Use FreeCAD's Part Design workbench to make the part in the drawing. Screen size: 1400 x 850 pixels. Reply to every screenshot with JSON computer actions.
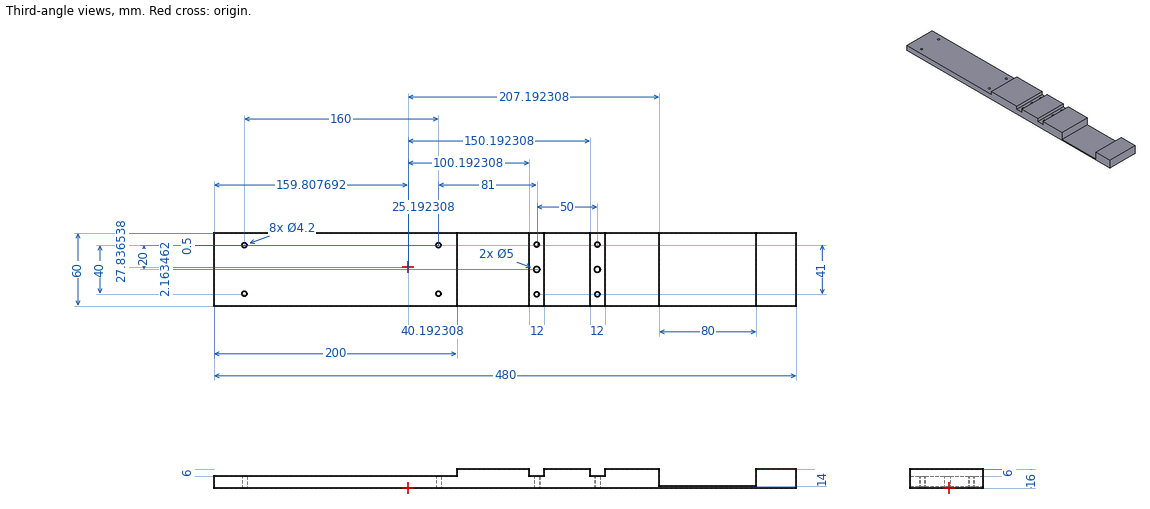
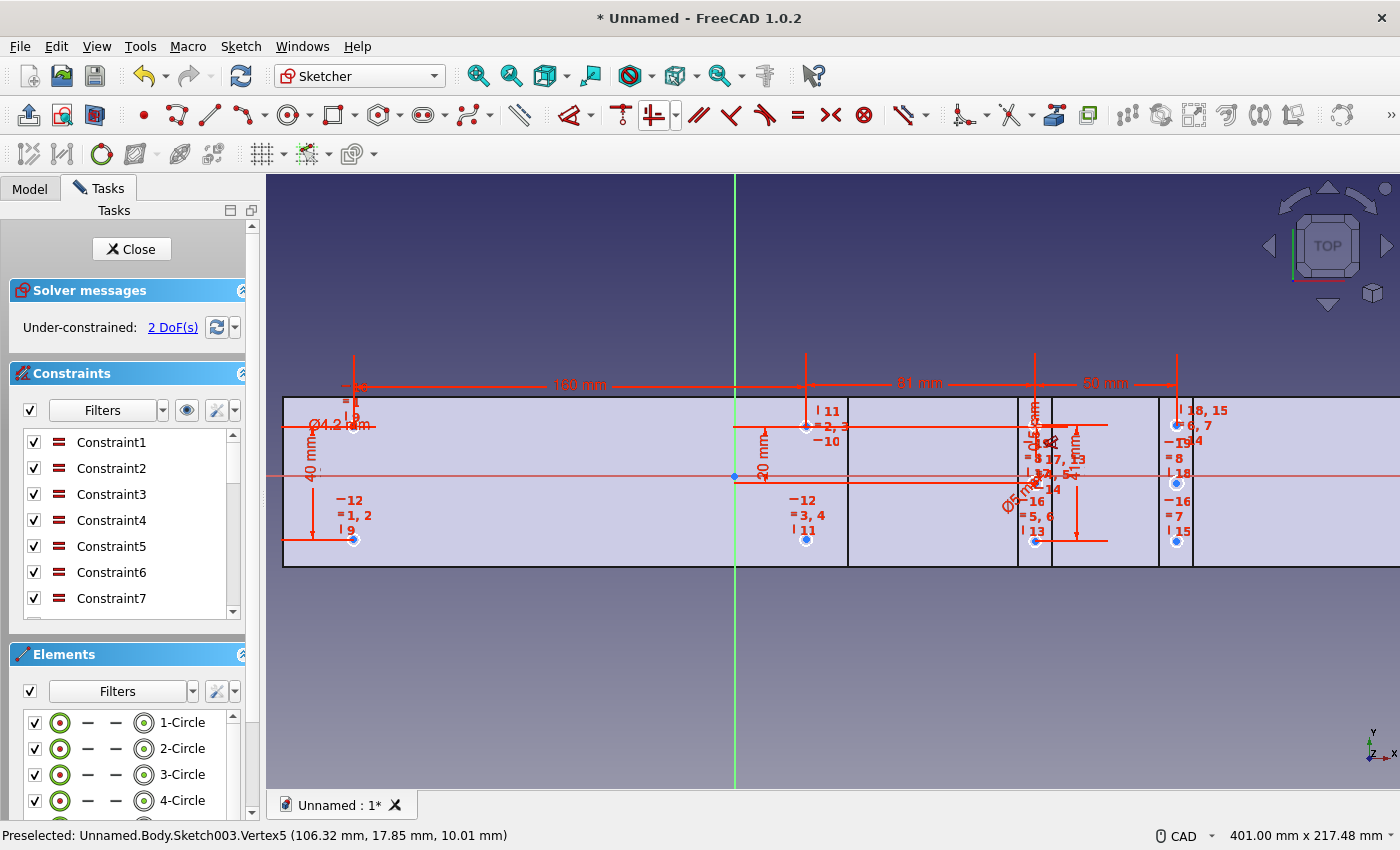
{"action": "scroll", "coordinate": [1035, 483], "scroll_direction": "up", "scroll_amount": 10}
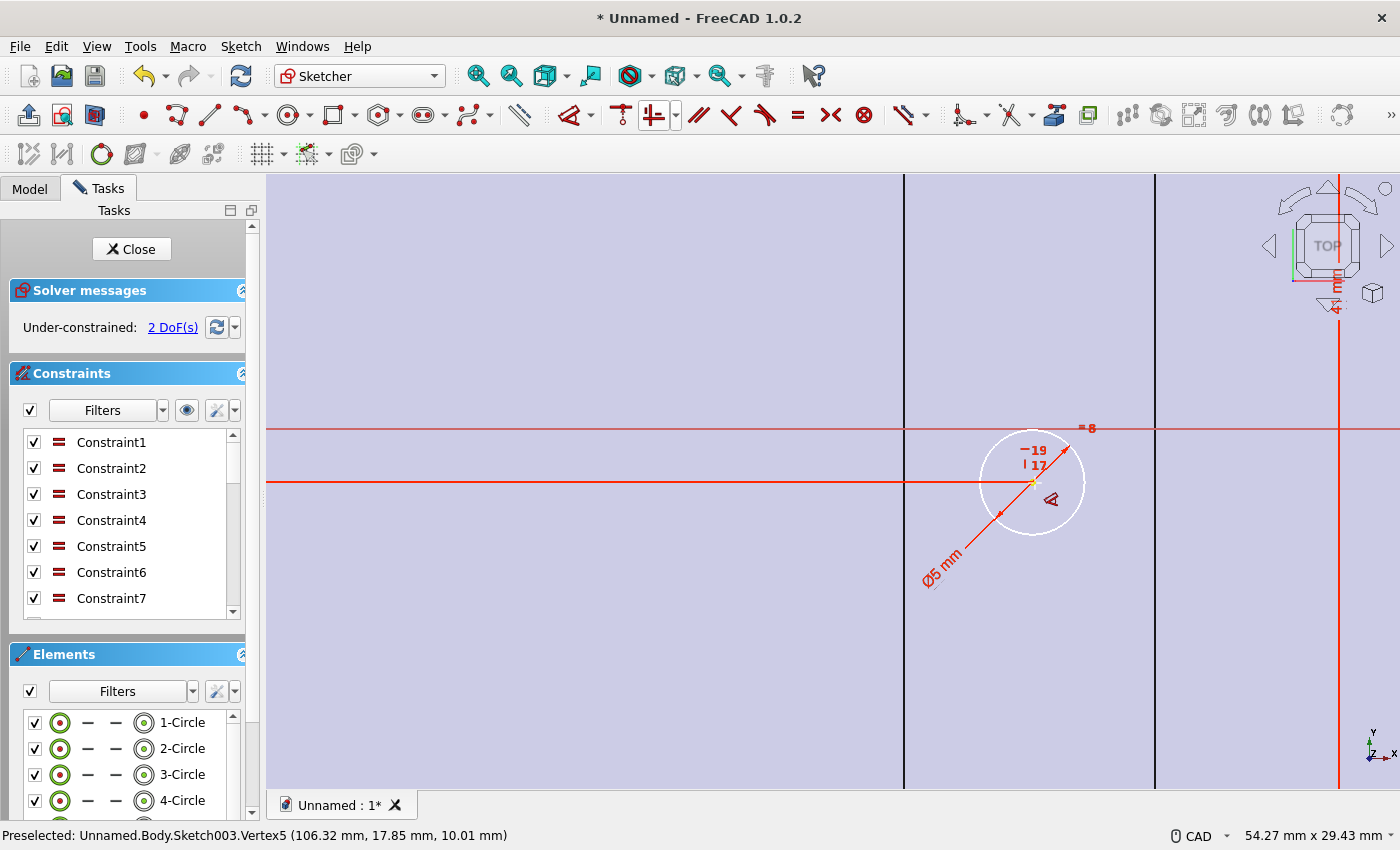
{"action": "left_click", "coordinate": [1032, 482]}
{"action": "left_click", "coordinate": [1066, 468]}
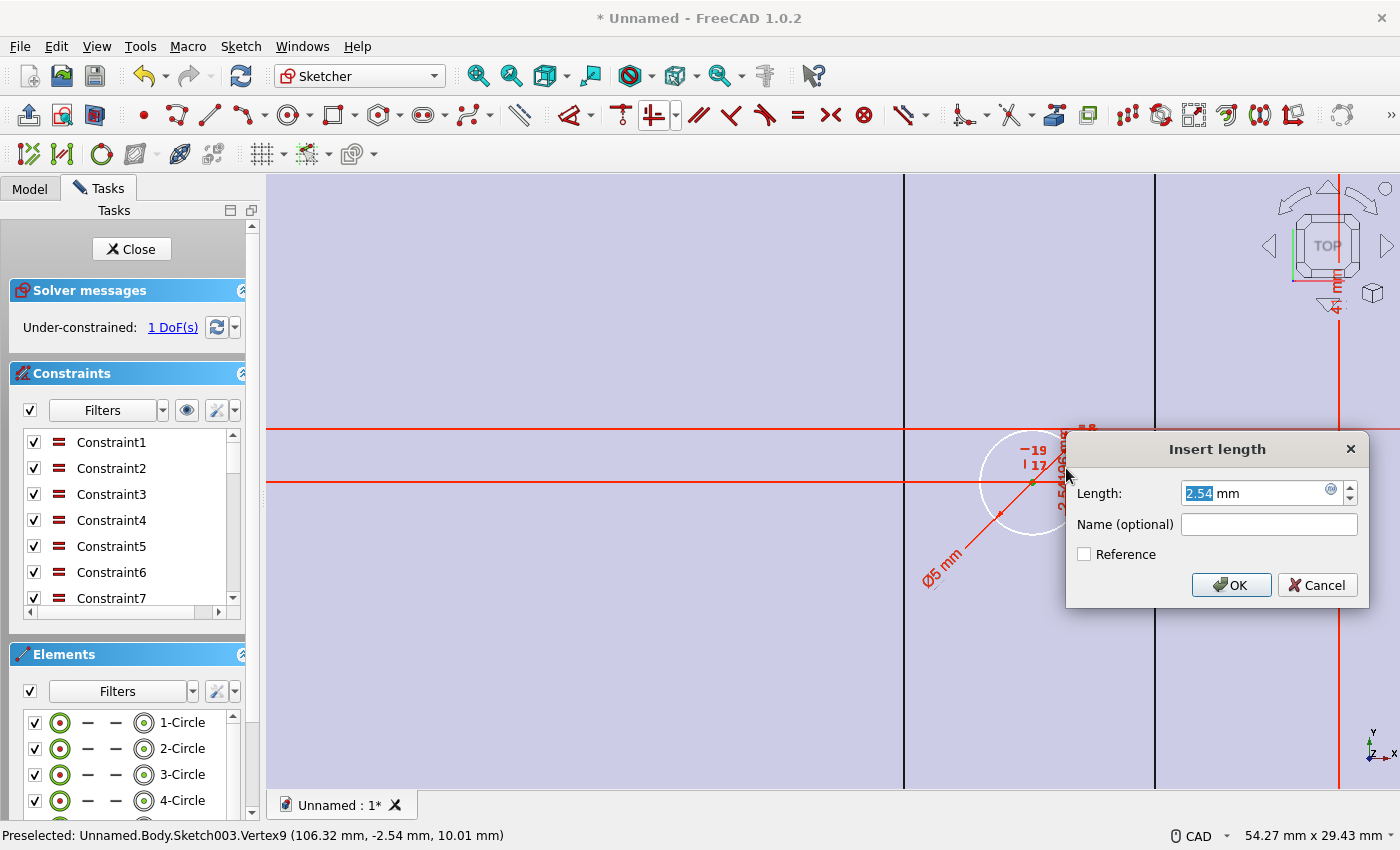
{"action": "type", "text": "2.163462"}
{"action": "key", "text": "Return"}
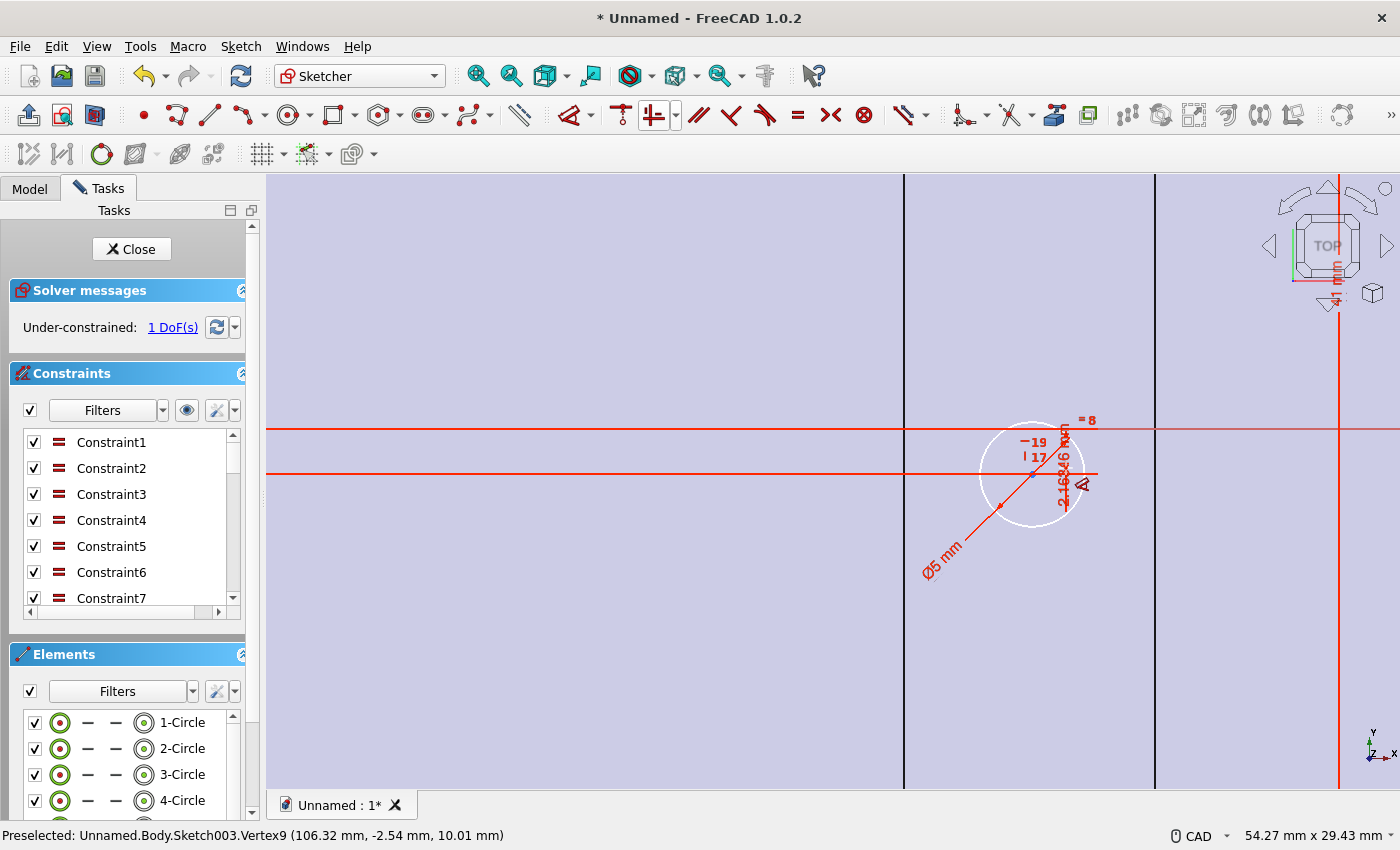
{"action": "scroll", "coordinate": [980, 482], "scroll_direction": "down", "scroll_amount": 11}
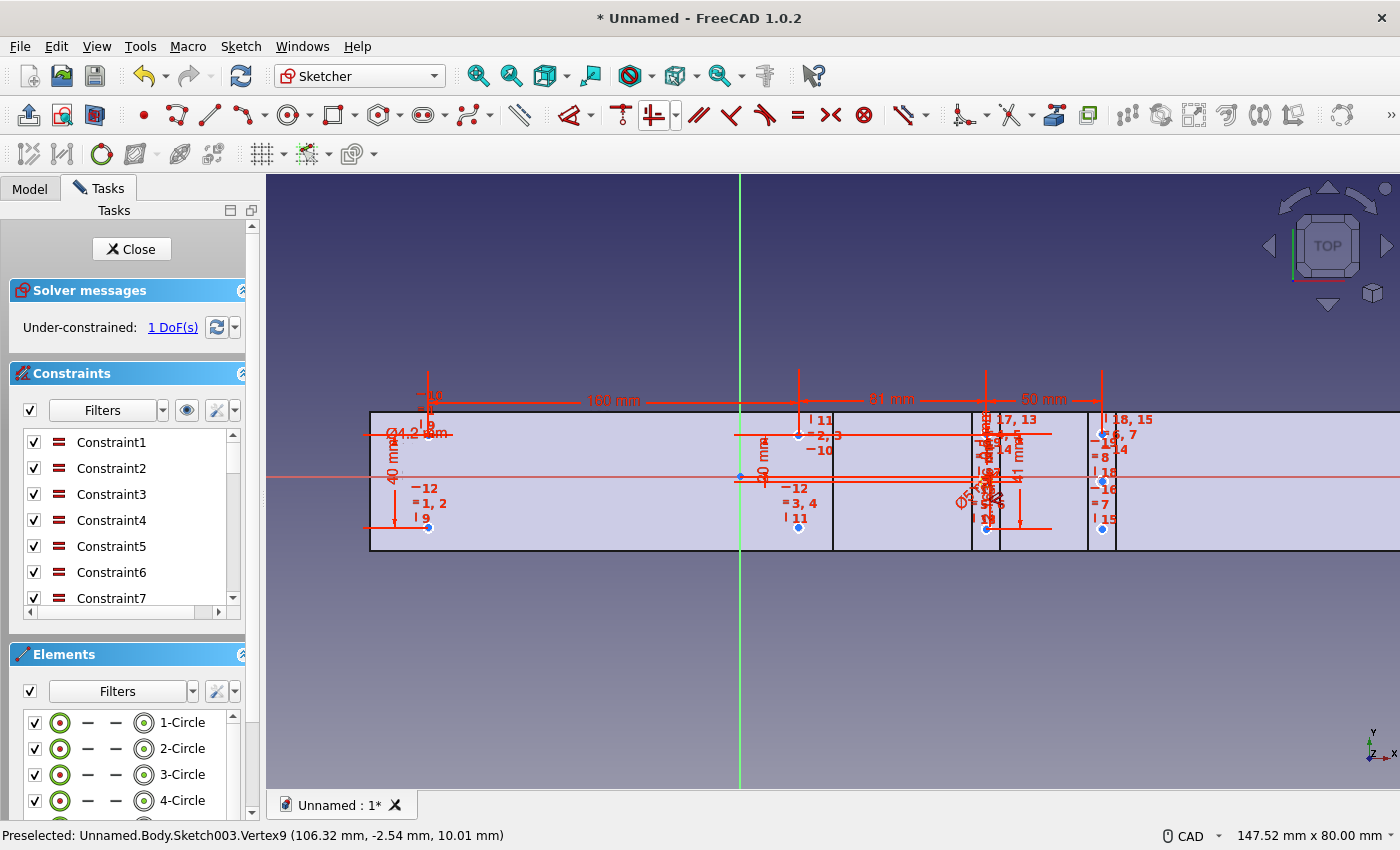
{"action": "left_click", "coordinate": [799, 435]}
{"action": "left_click", "coordinate": [770, 401]}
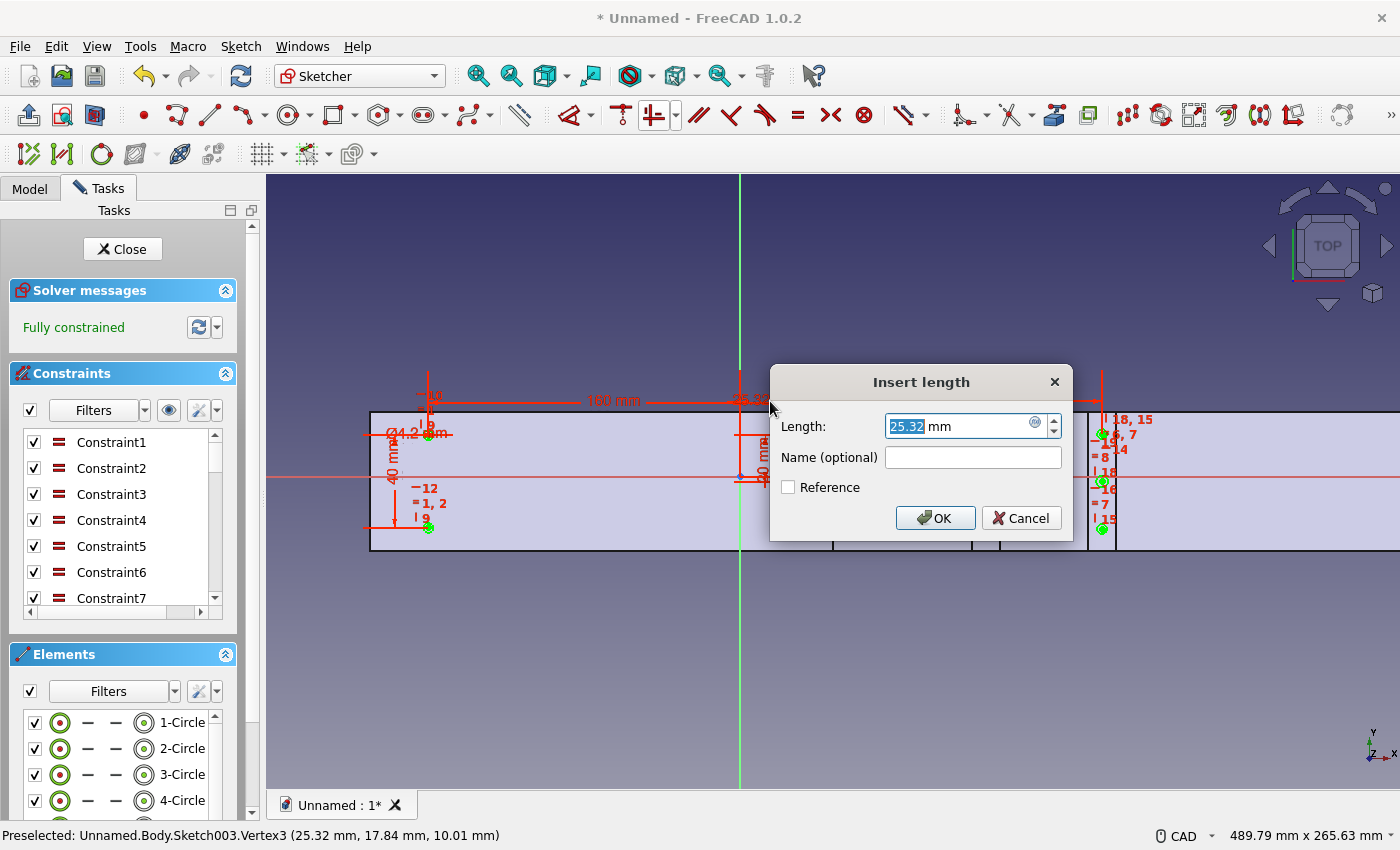
{"action": "type", "text": "25.192308"}
{"action": "key", "text": "Return"}
{"action": "key", "text": "Escape"}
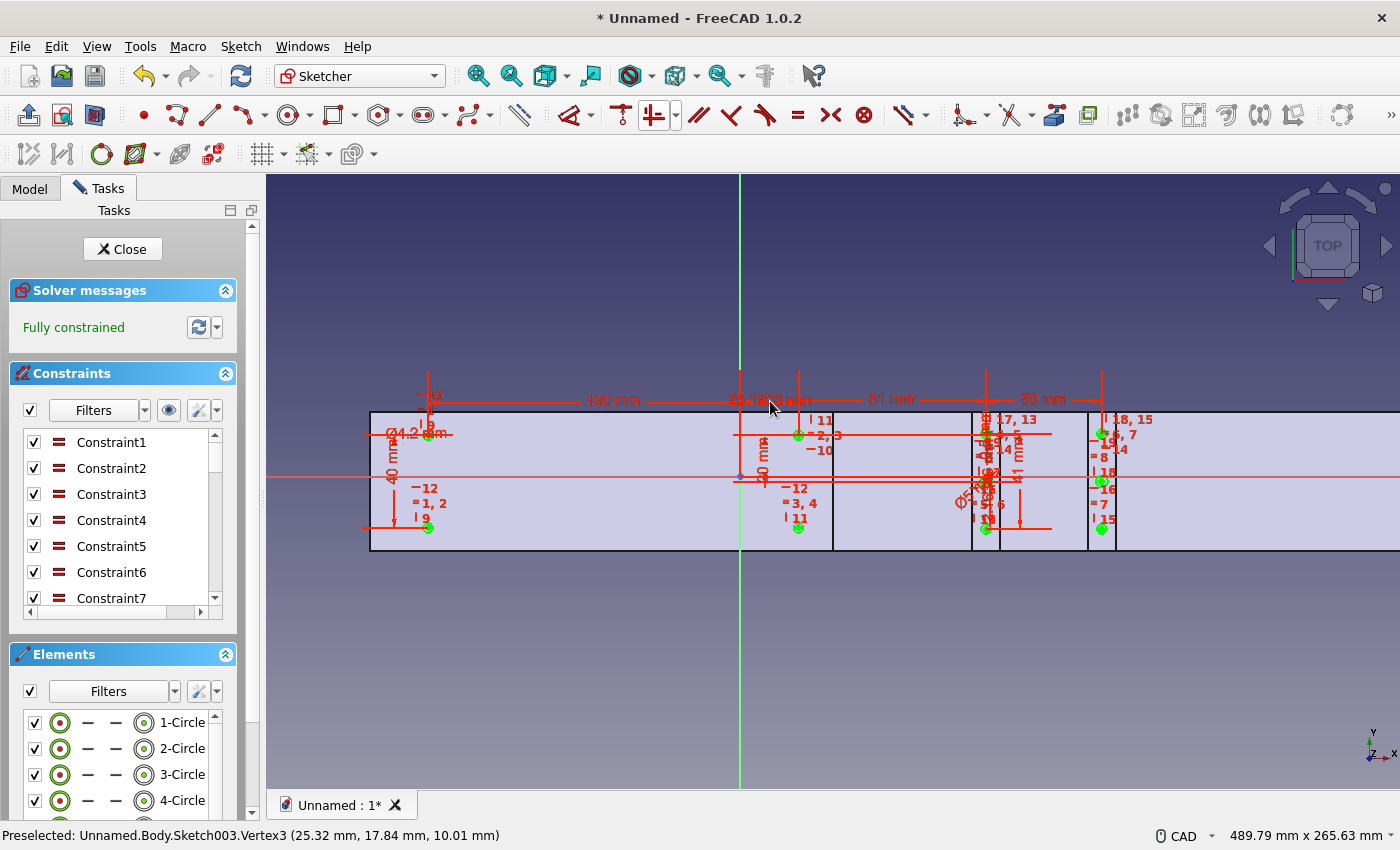
{"action": "left_click", "coordinate": [123, 249]}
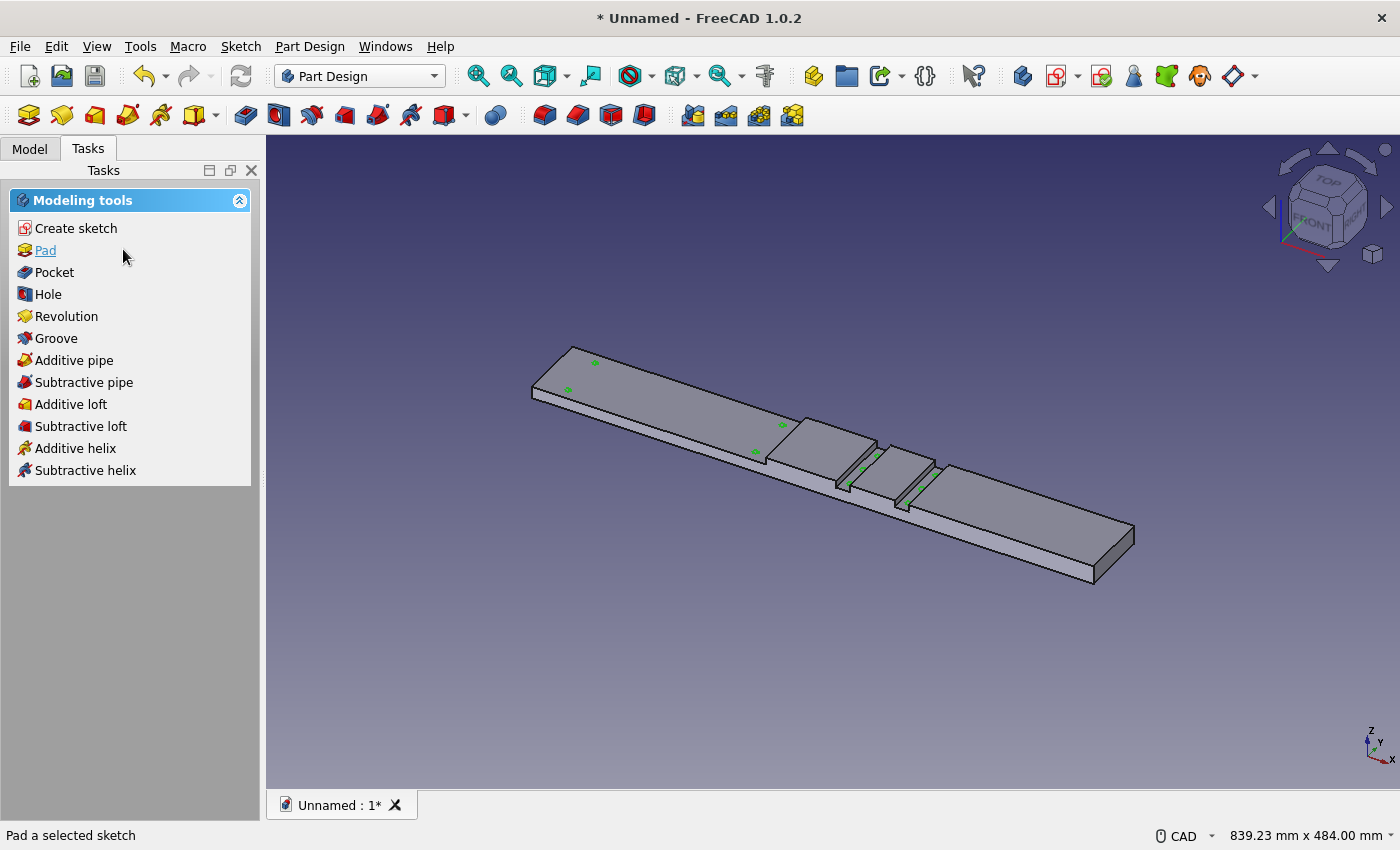
{"action": "left_click", "coordinate": [246, 116]}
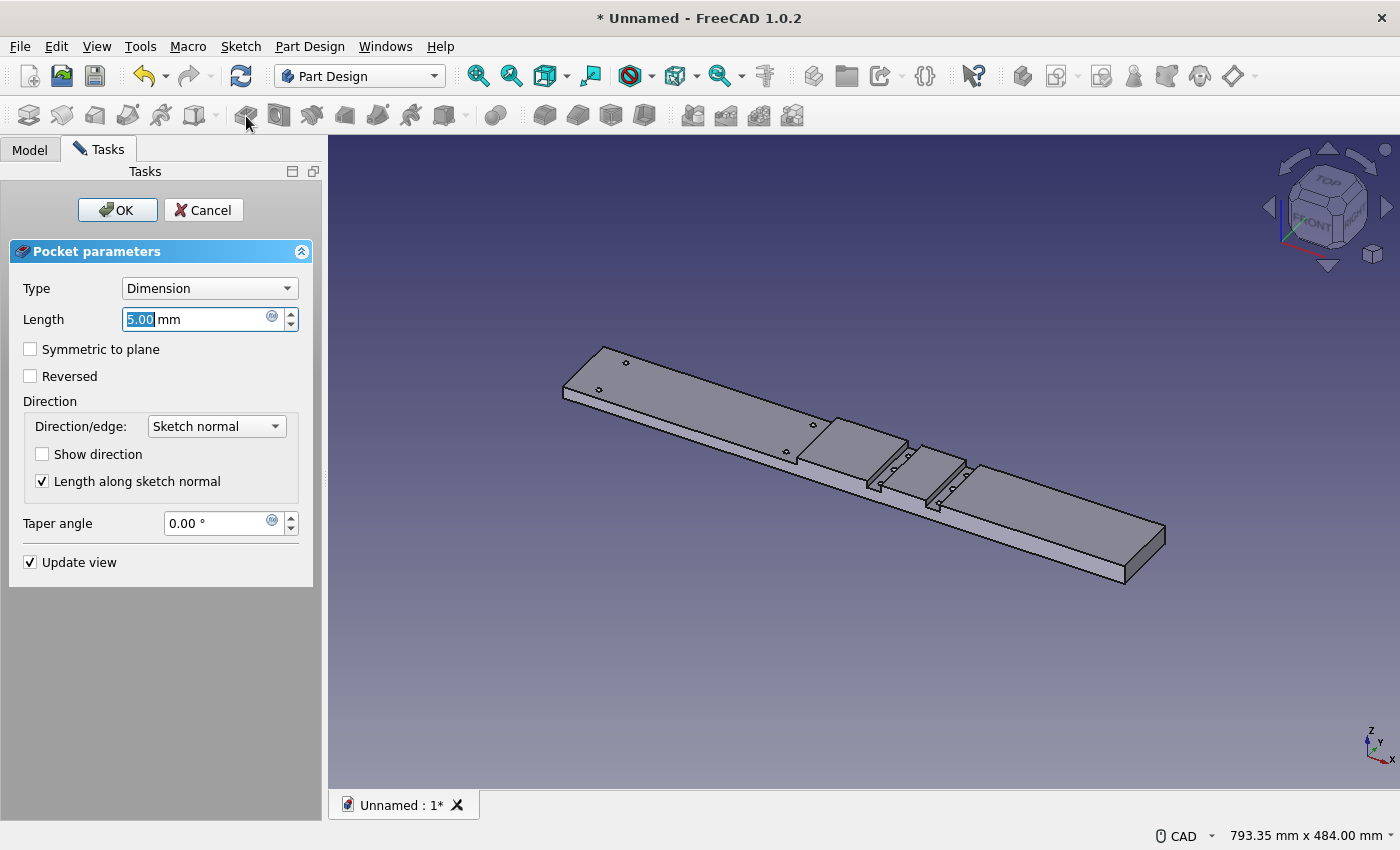
{"action": "left_click", "coordinate": [210, 288]}